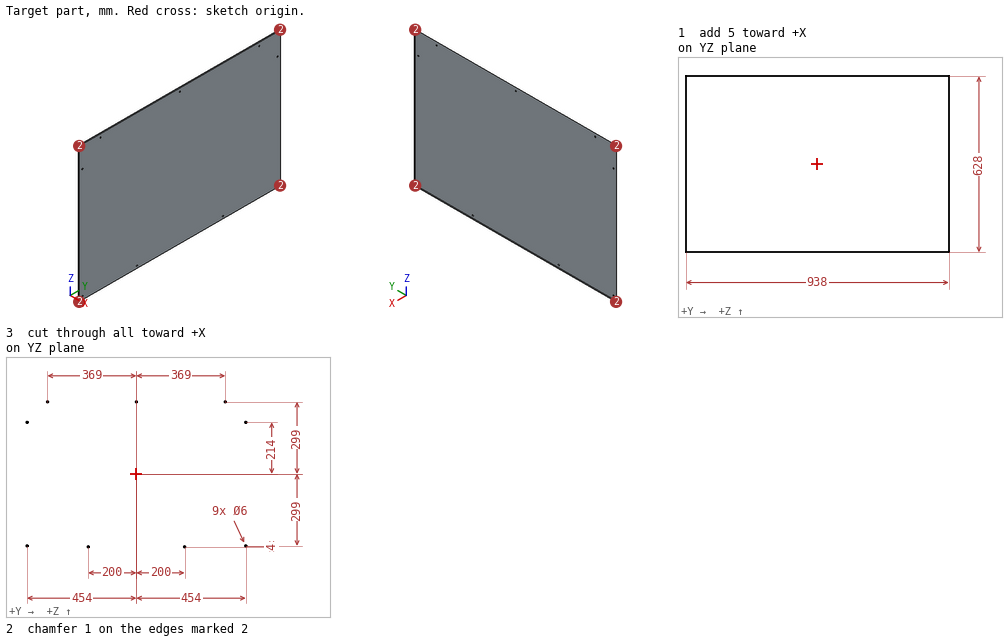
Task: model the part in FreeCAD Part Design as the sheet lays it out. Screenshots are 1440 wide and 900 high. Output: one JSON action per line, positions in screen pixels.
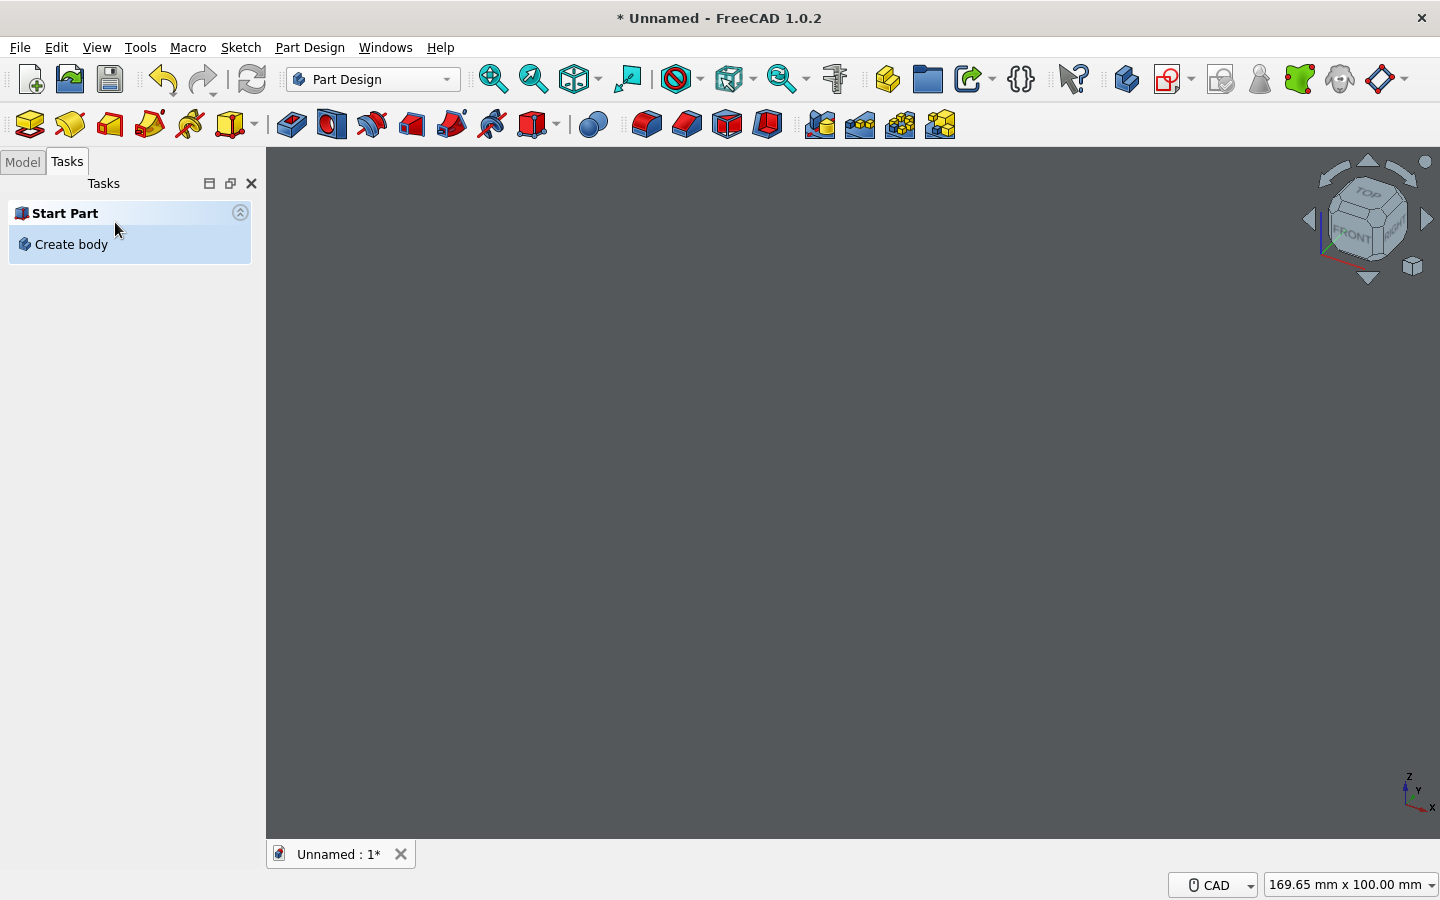
{"action": "key", "text": "v f"}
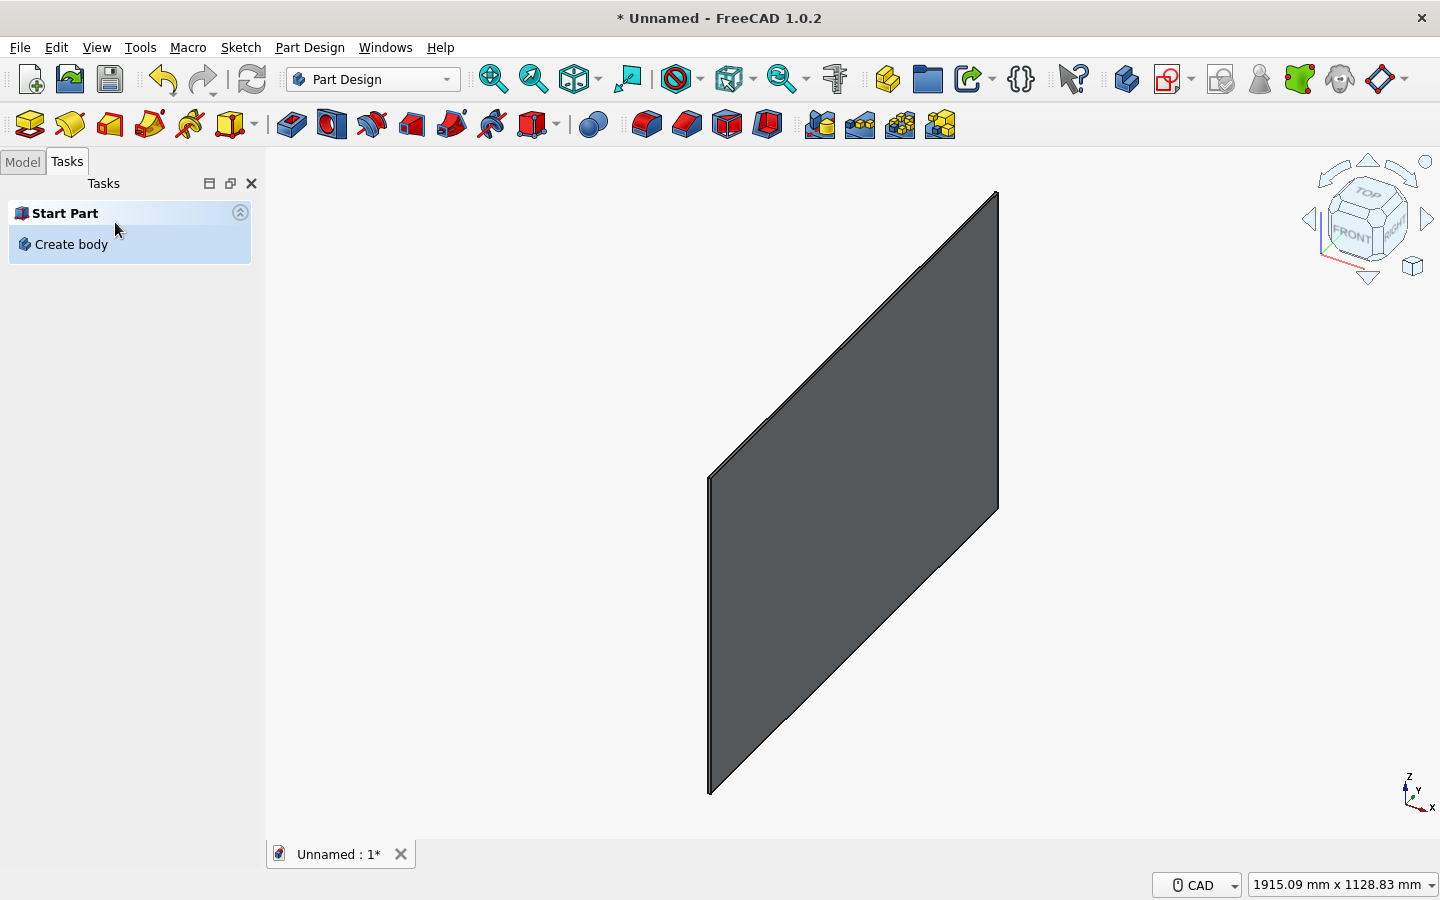
{"action": "scroll", "coordinate": [997, 192], "scroll_direction": "up", "scroll_amount": 13}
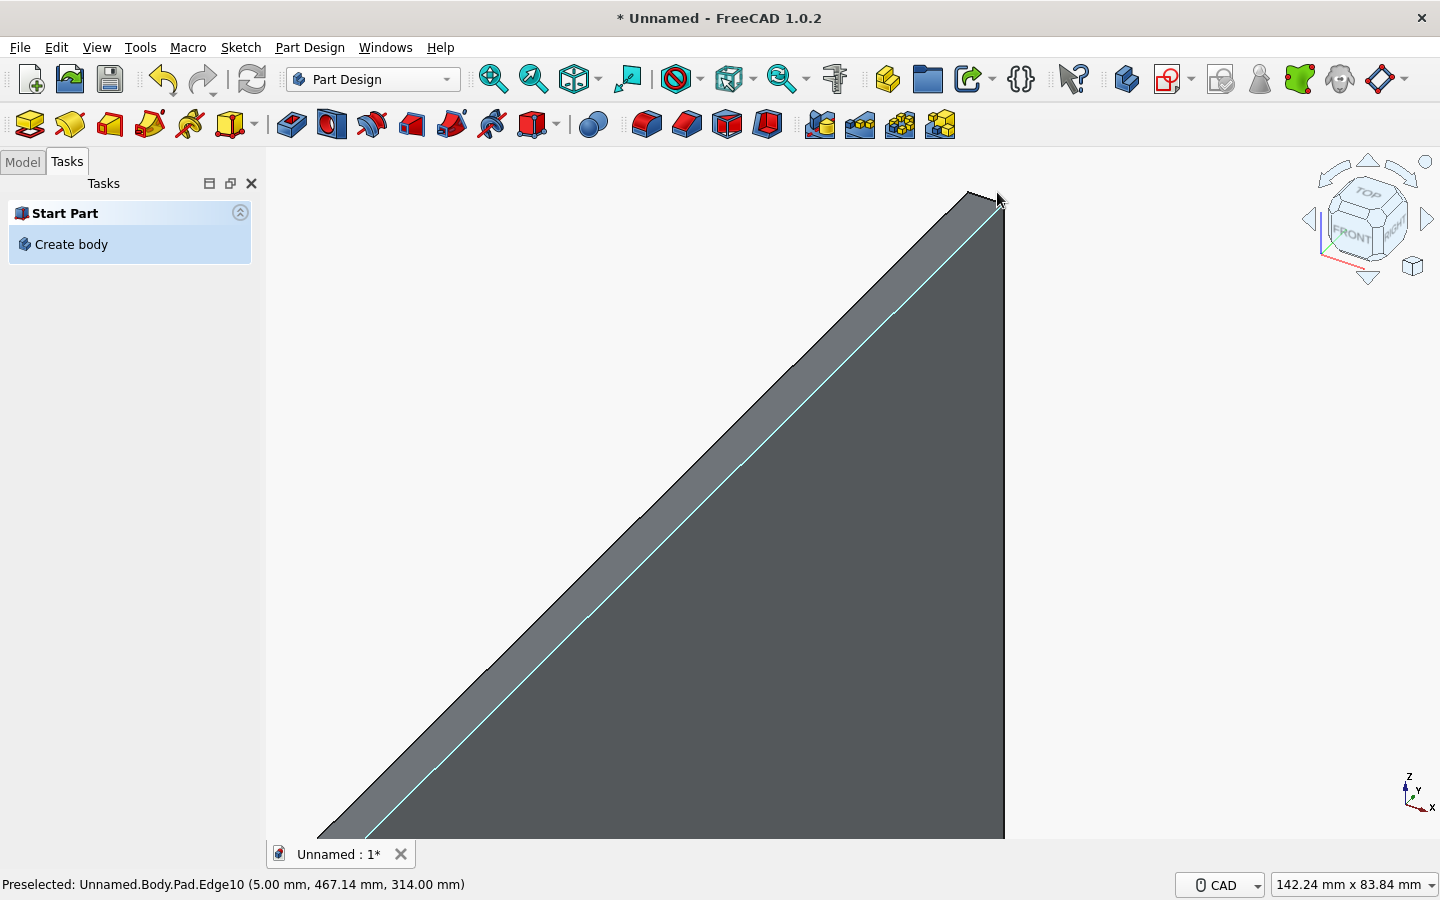
{"action": "key", "text": "v f"}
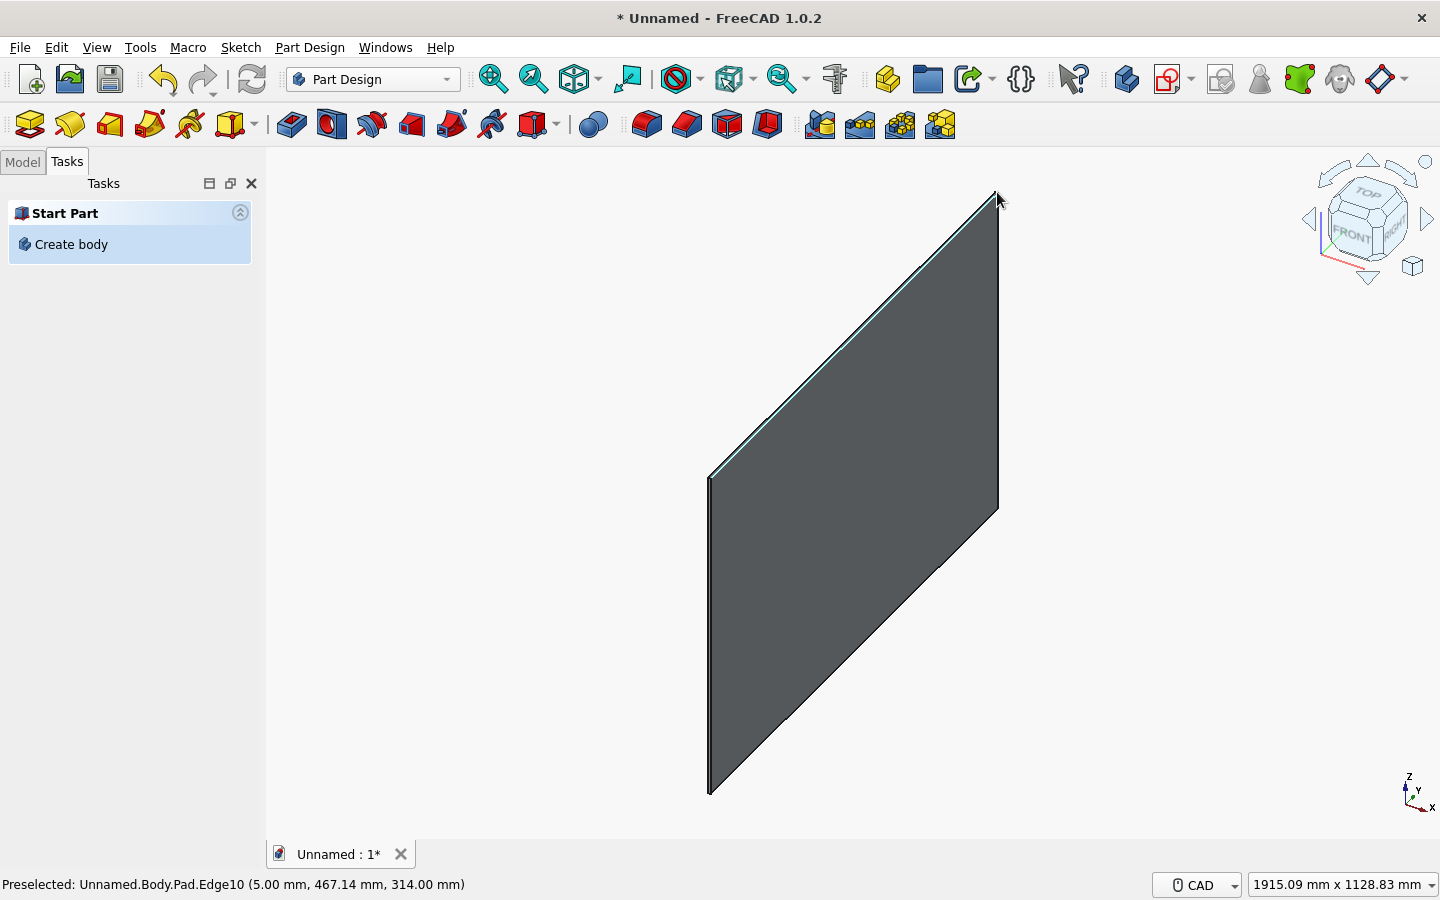
{"action": "key", "text": "0"}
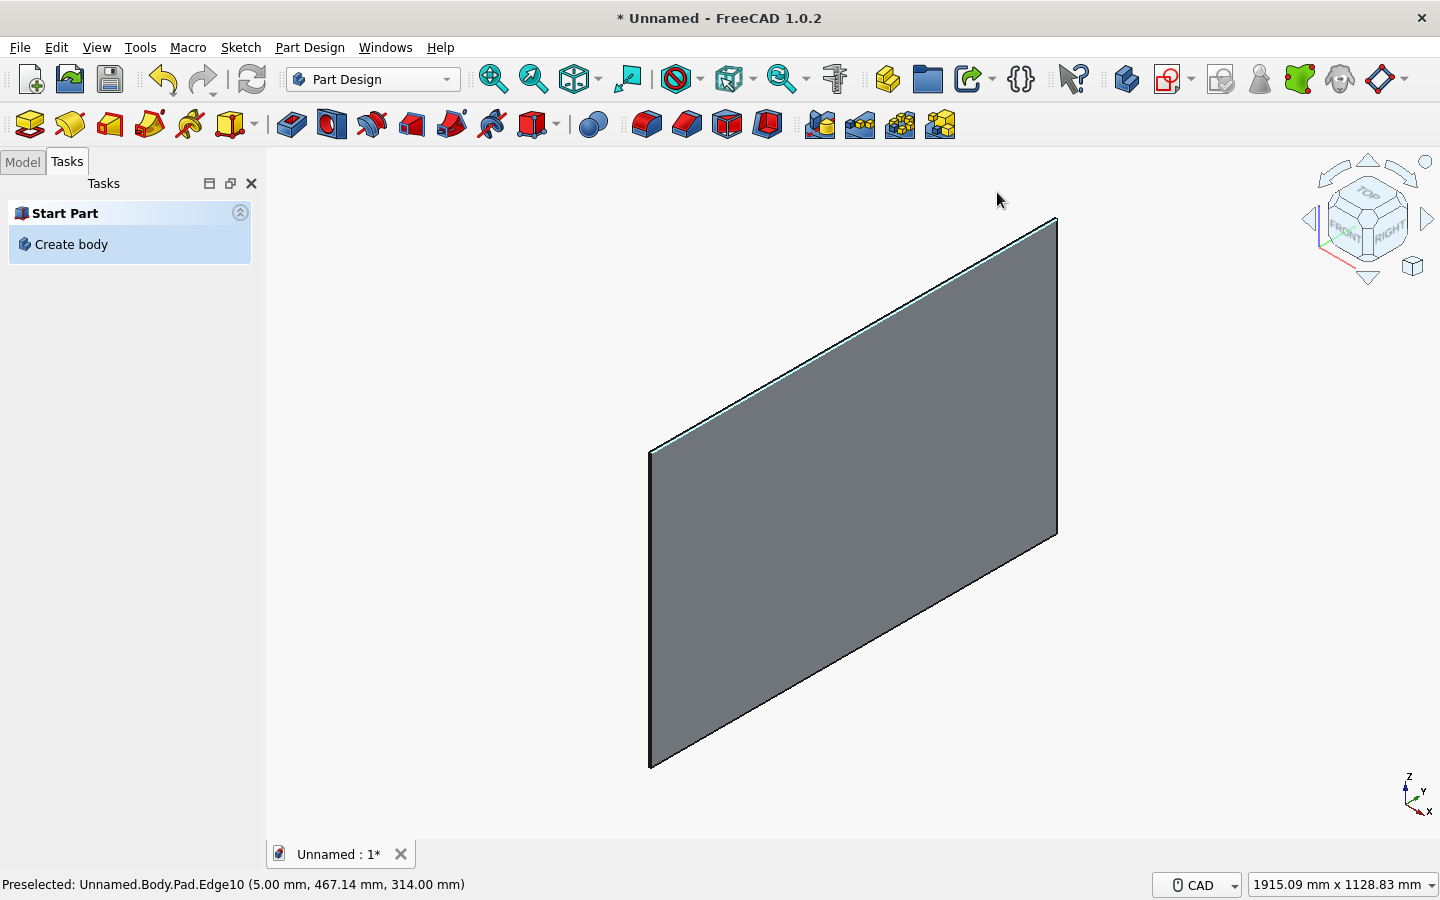
{"action": "scroll", "coordinate": [1056, 217], "scroll_direction": "up", "scroll_amount": 13}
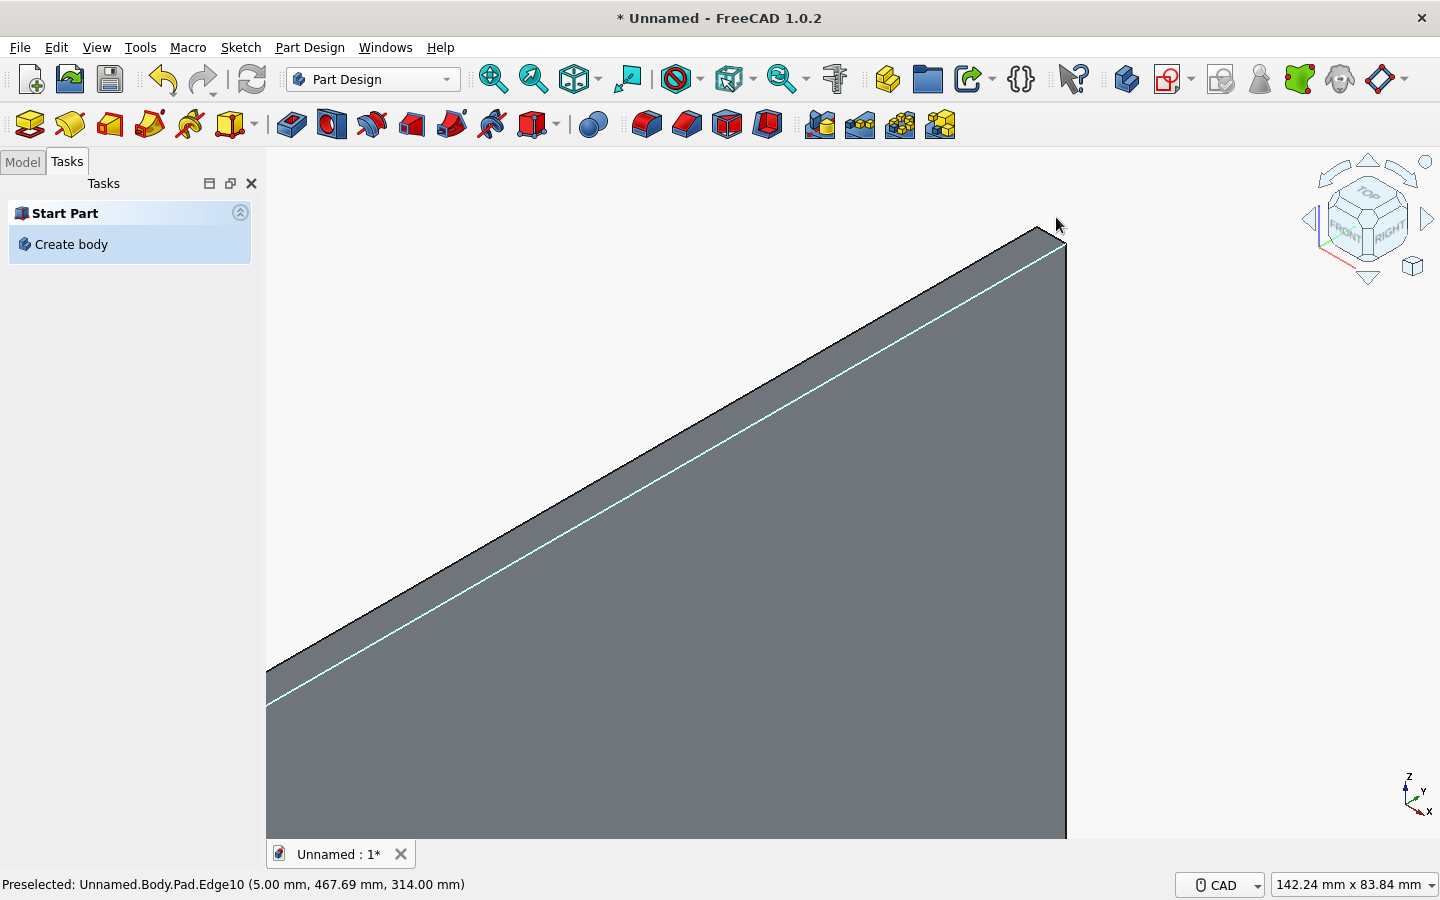
{"action": "left_click", "coordinate": [494, 80]}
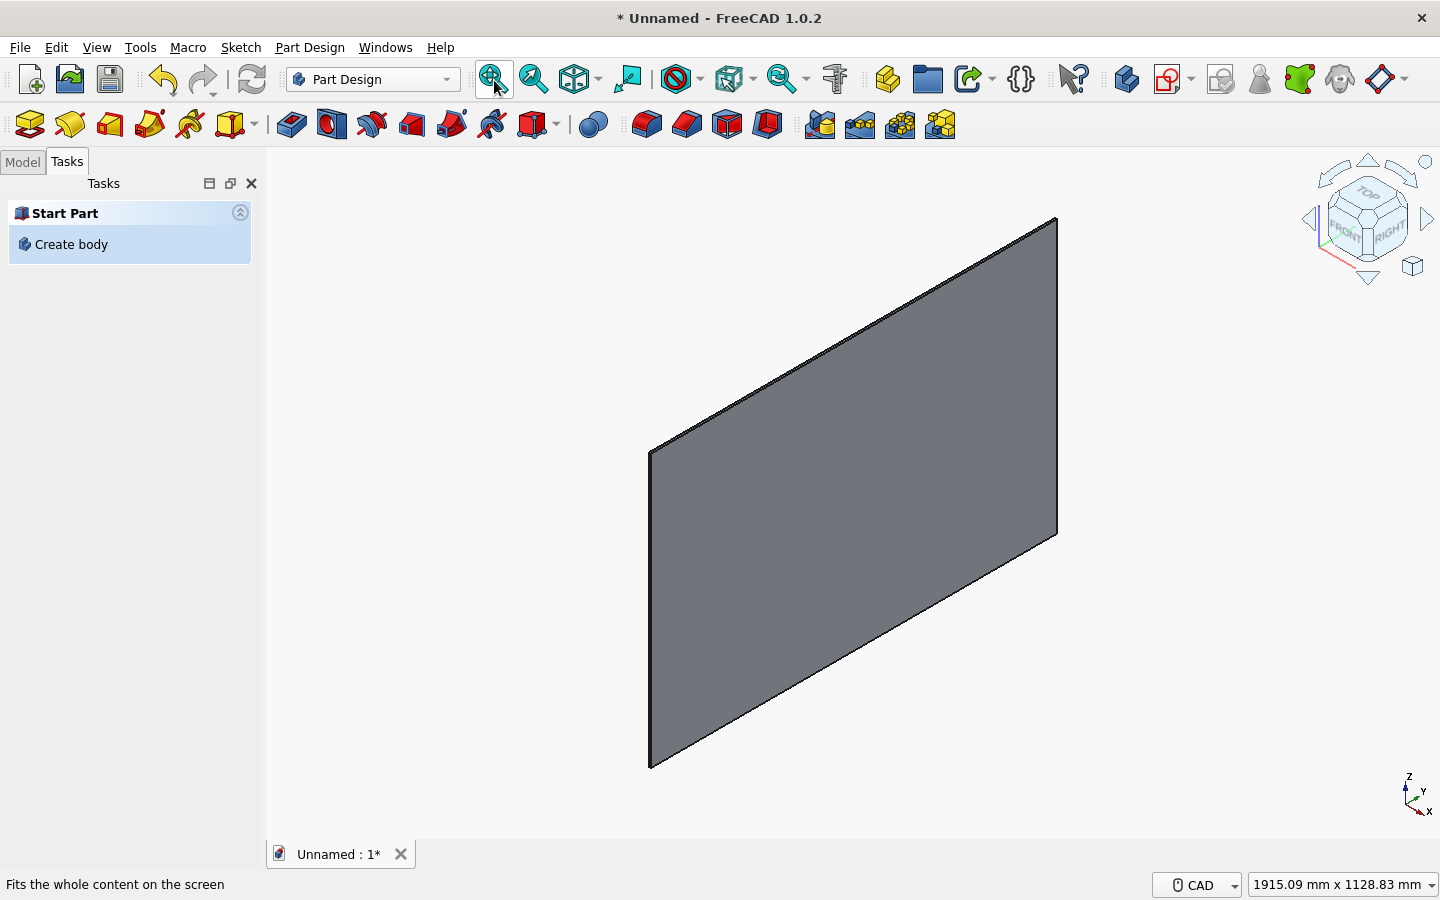
{"action": "key", "text": "2"}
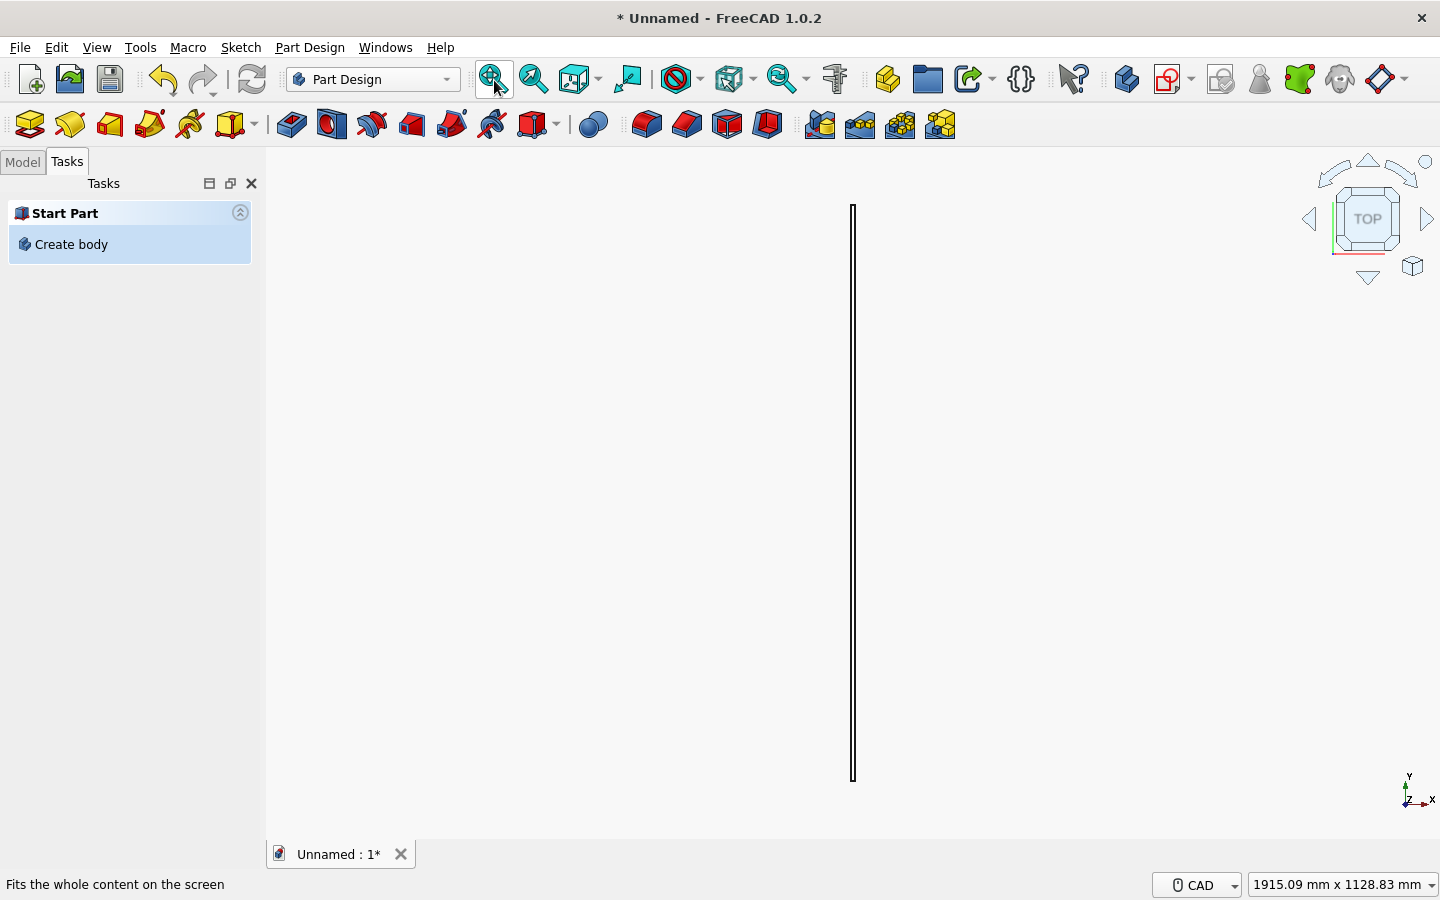
{"action": "scroll", "coordinate": [853, 204], "scroll_direction": "up", "scroll_amount": 13}